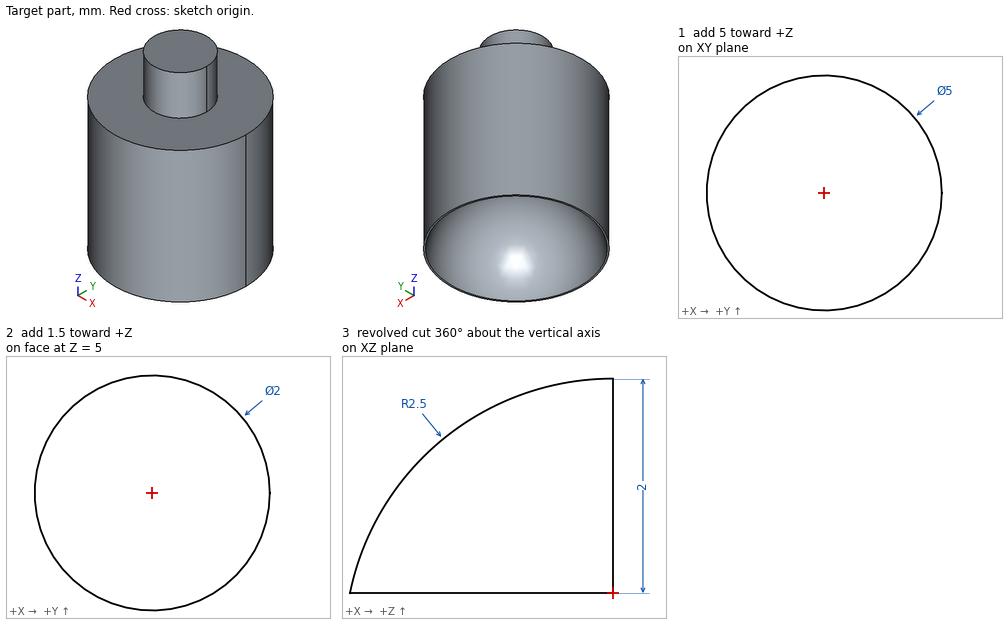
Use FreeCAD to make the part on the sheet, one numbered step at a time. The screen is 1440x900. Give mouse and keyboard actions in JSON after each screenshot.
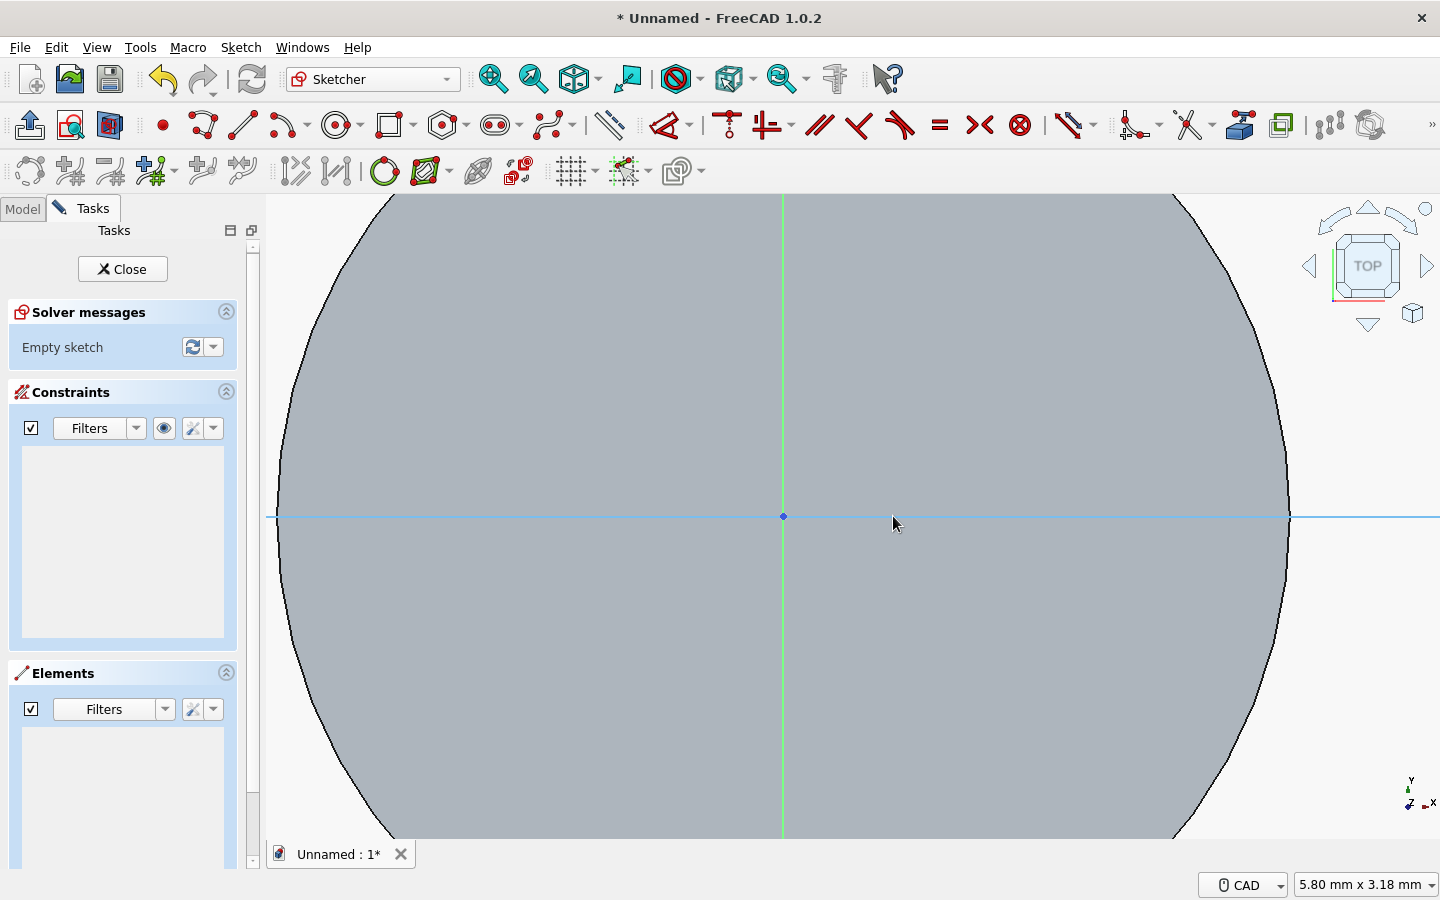
{"action": "left_click", "coordinate": [336, 126]}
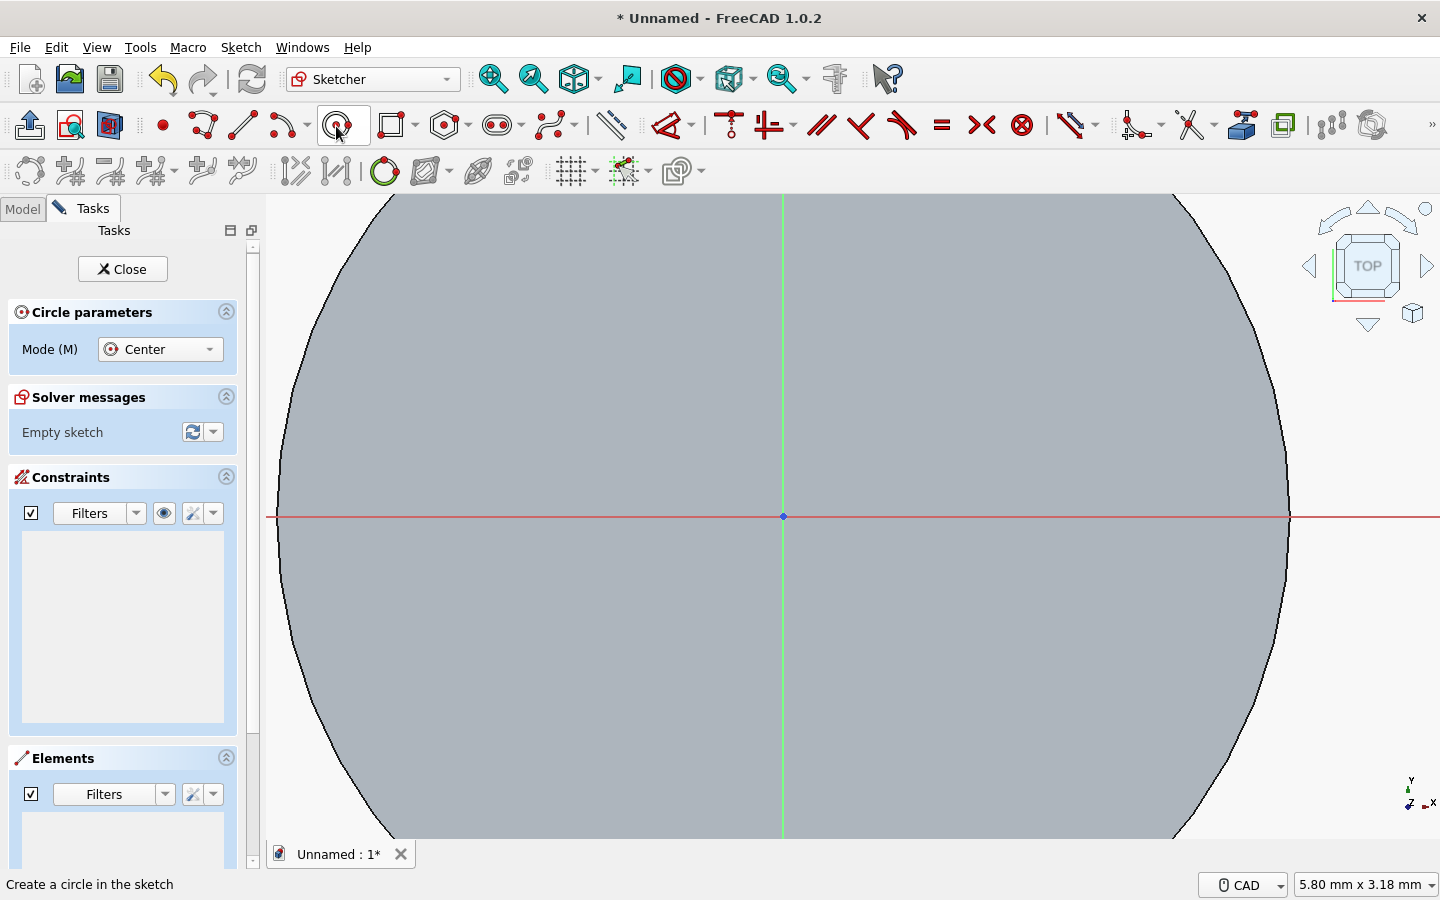
{"action": "left_click", "coordinate": [783, 516]}
{"action": "mouse_move", "coordinate": [927, 373]}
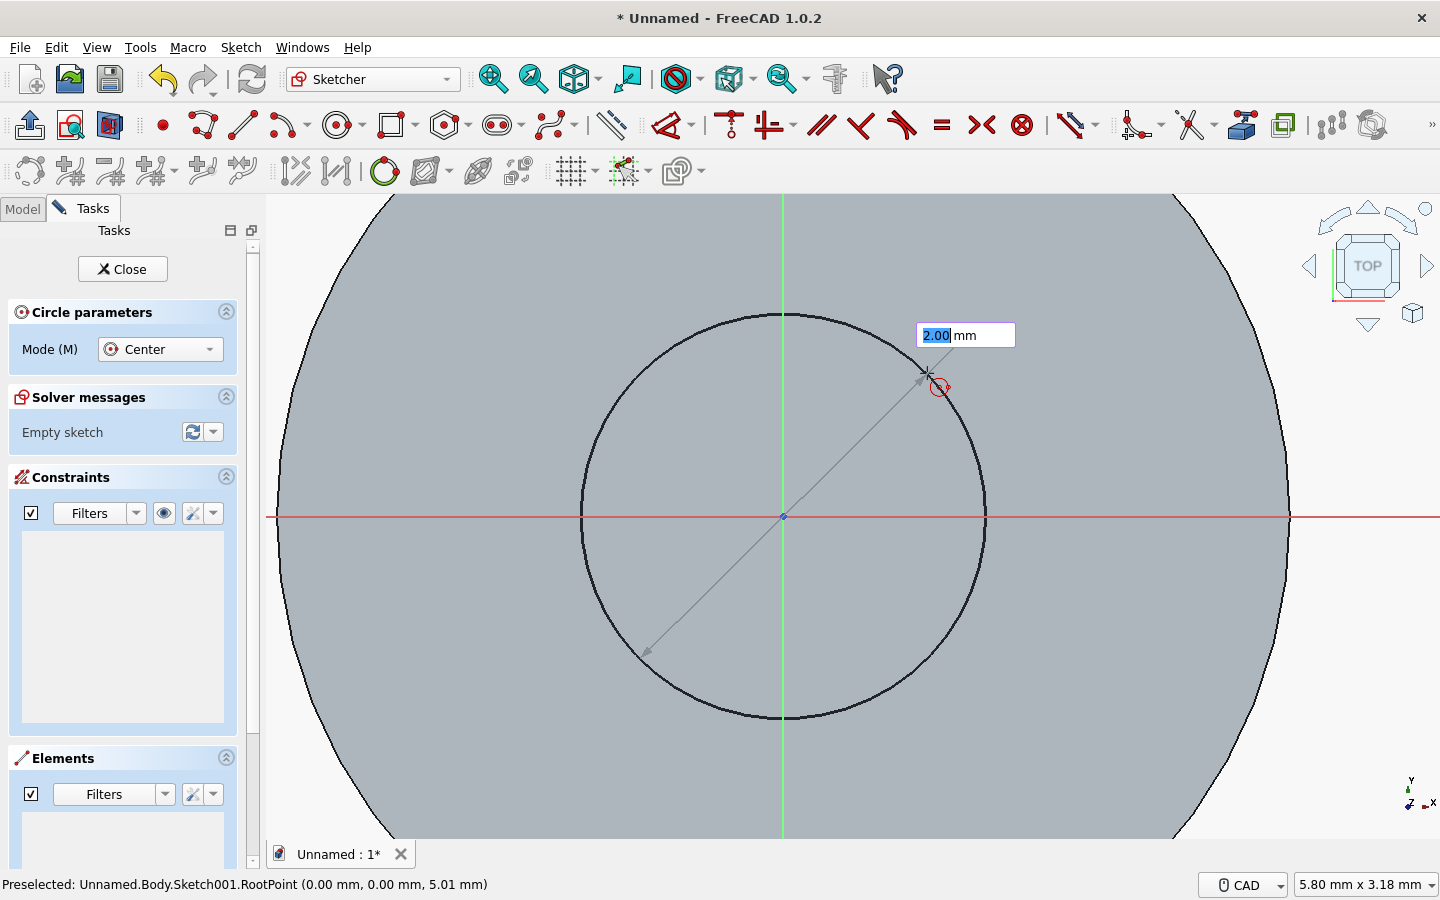
{"action": "type", "text": "2"}
{"action": "key", "text": "Return"}
{"action": "key", "text": "Escape"}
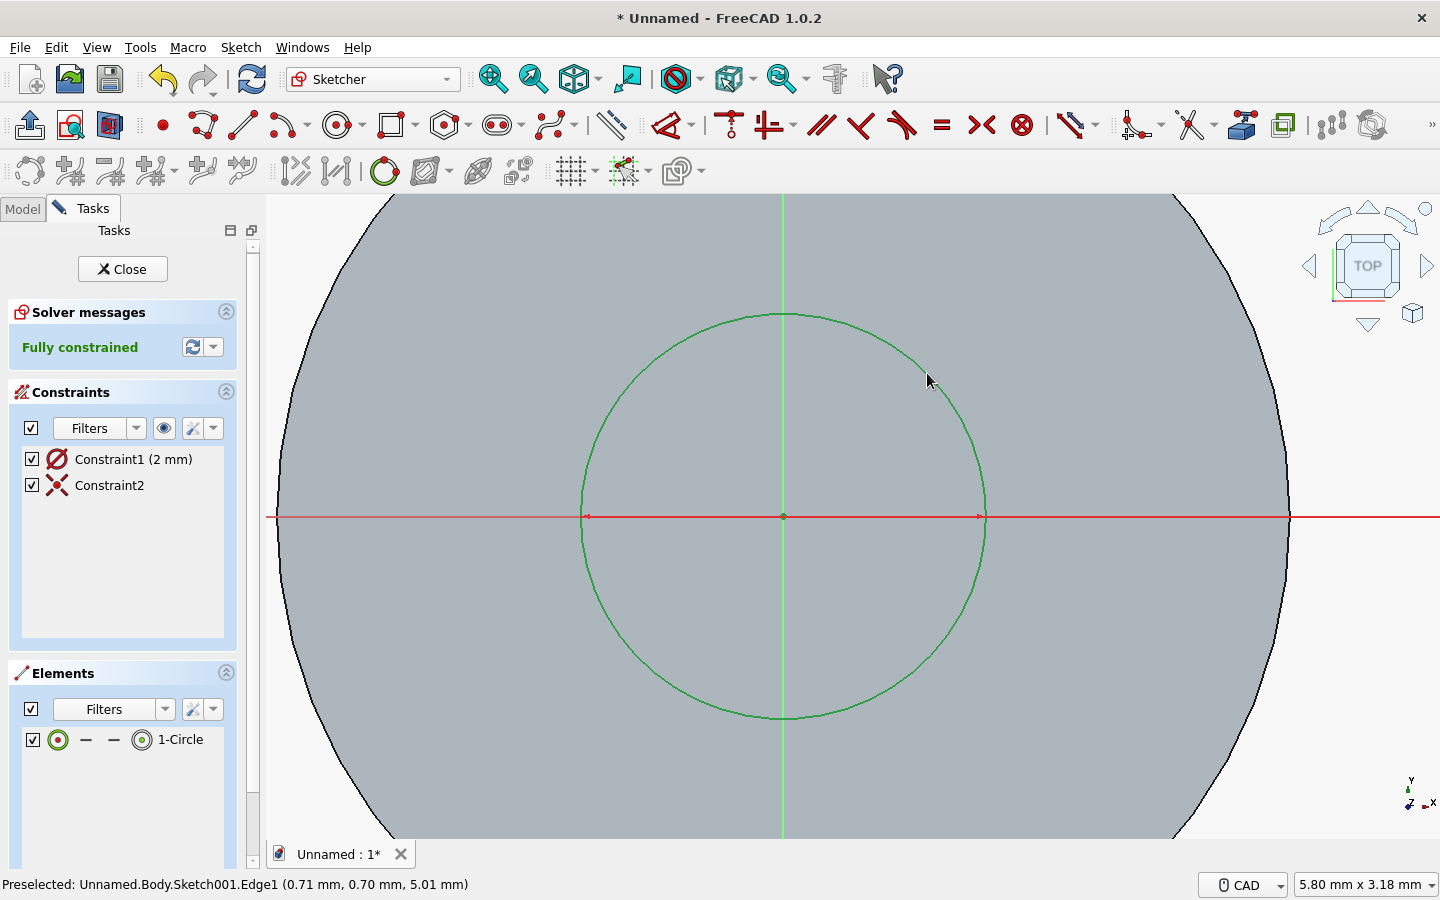
{"action": "left_click", "coordinate": [123, 269]}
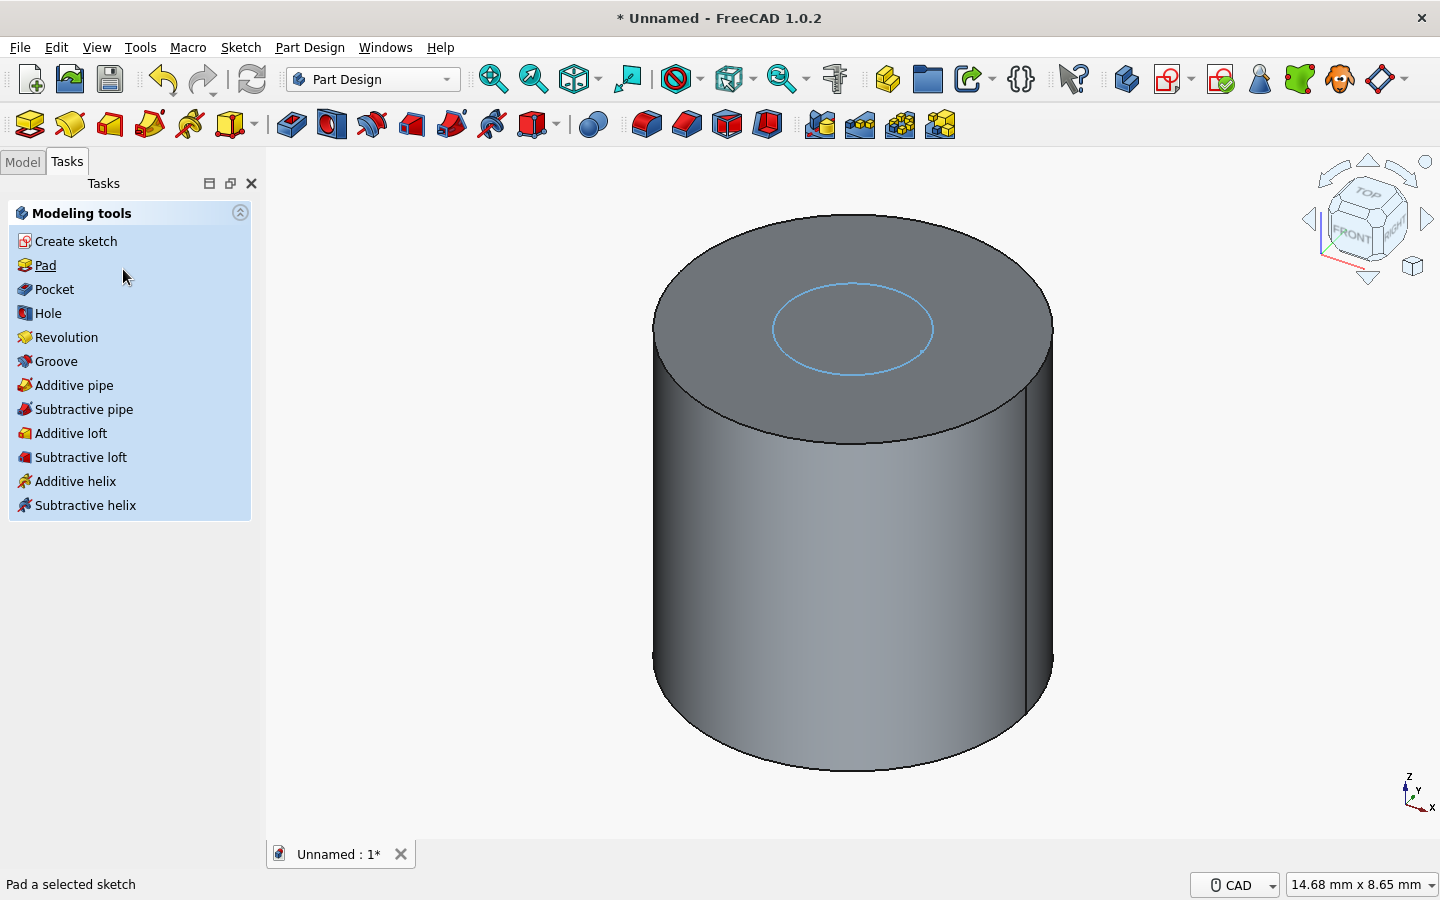
{"action": "left_click", "coordinate": [30, 124]}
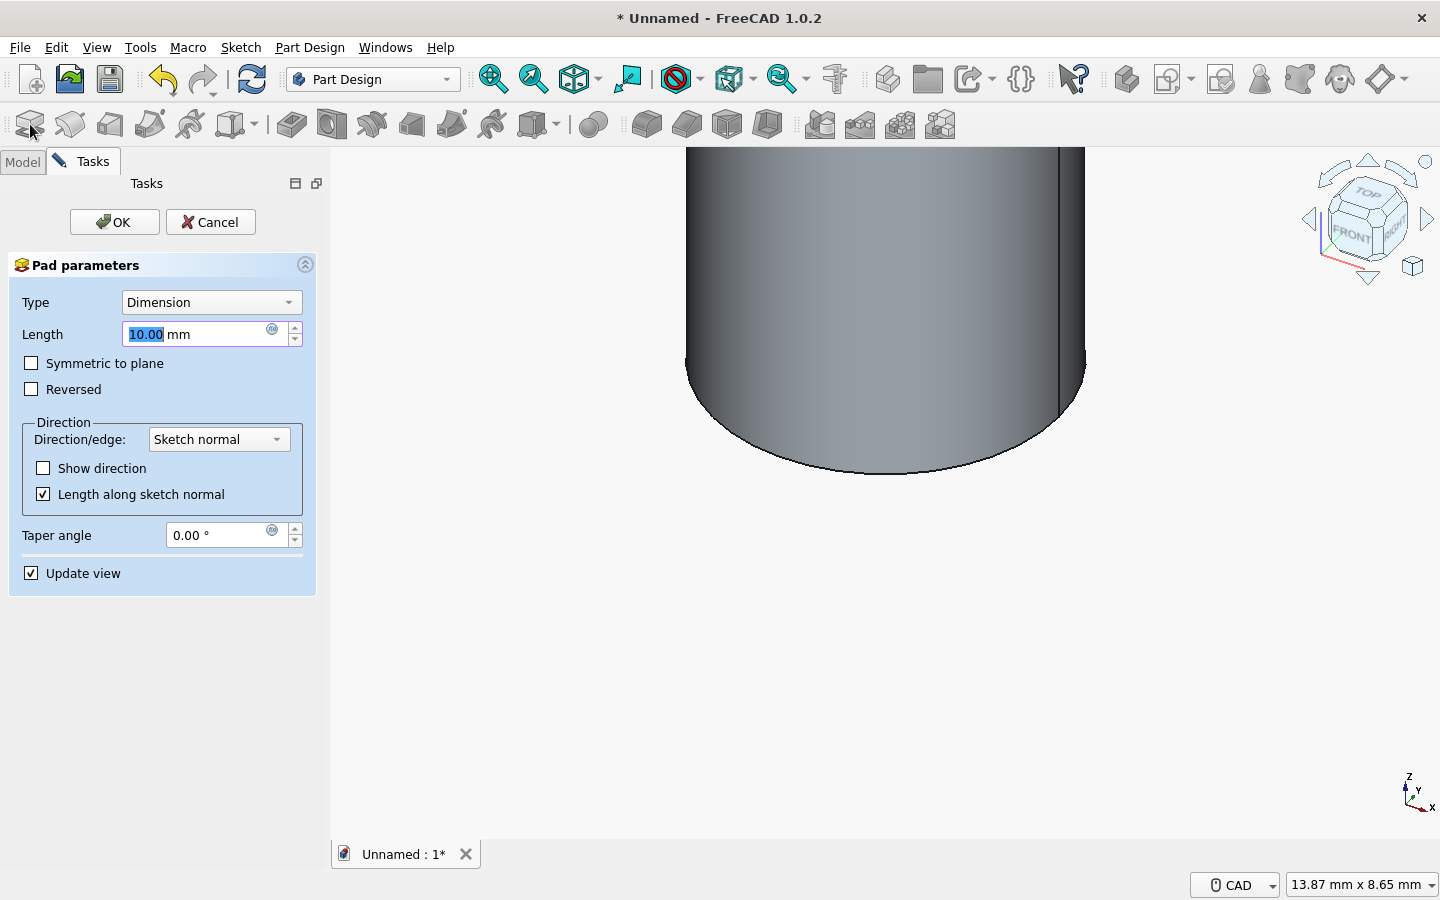
{"action": "type", "text": "1.5"}
{"action": "key", "text": "Tab"}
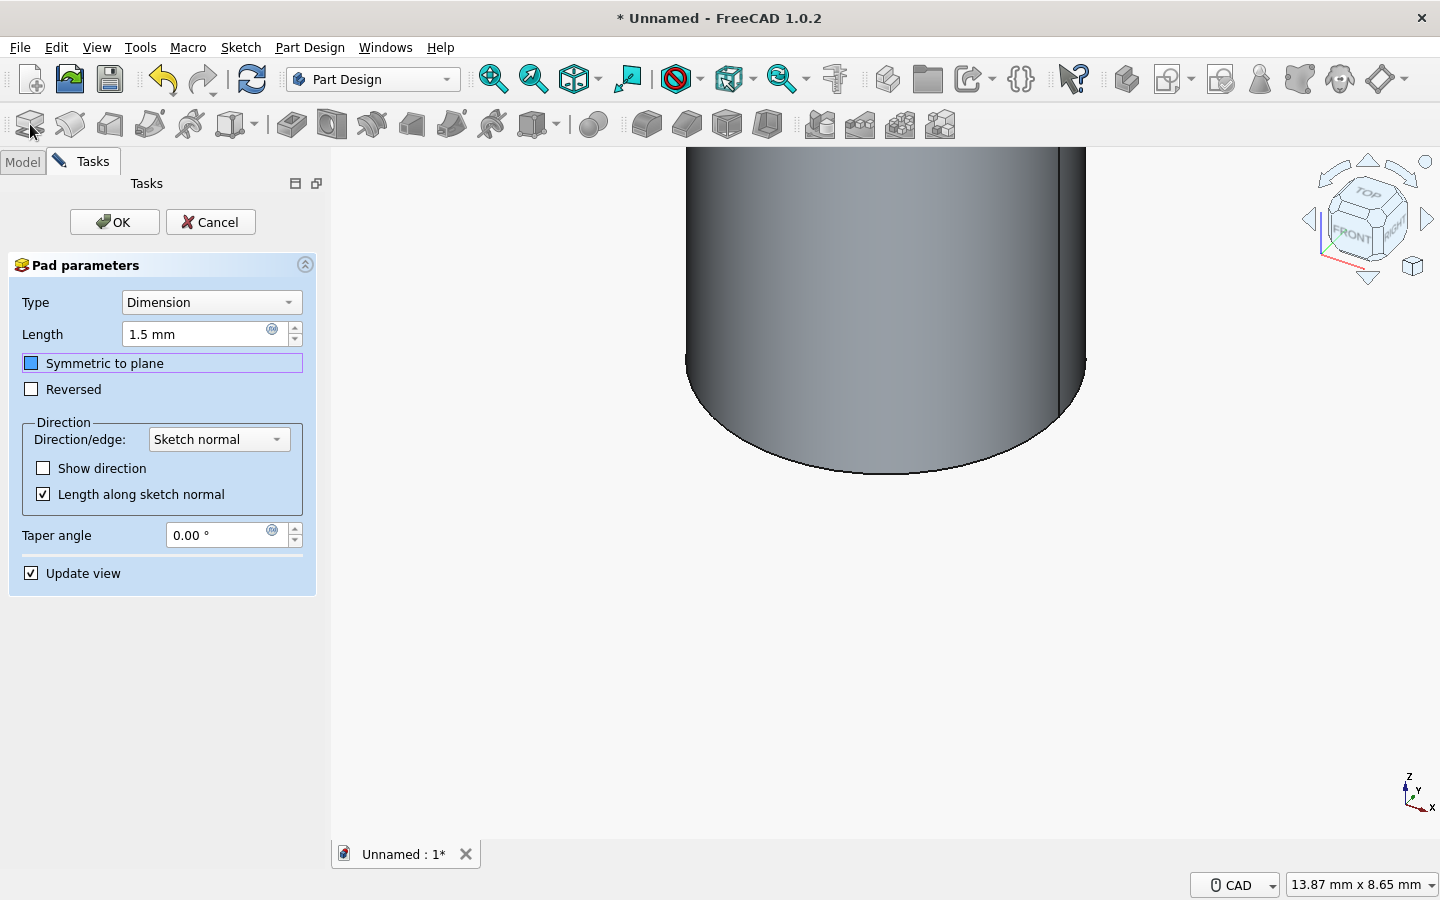
{"action": "left_click", "coordinate": [115, 222]}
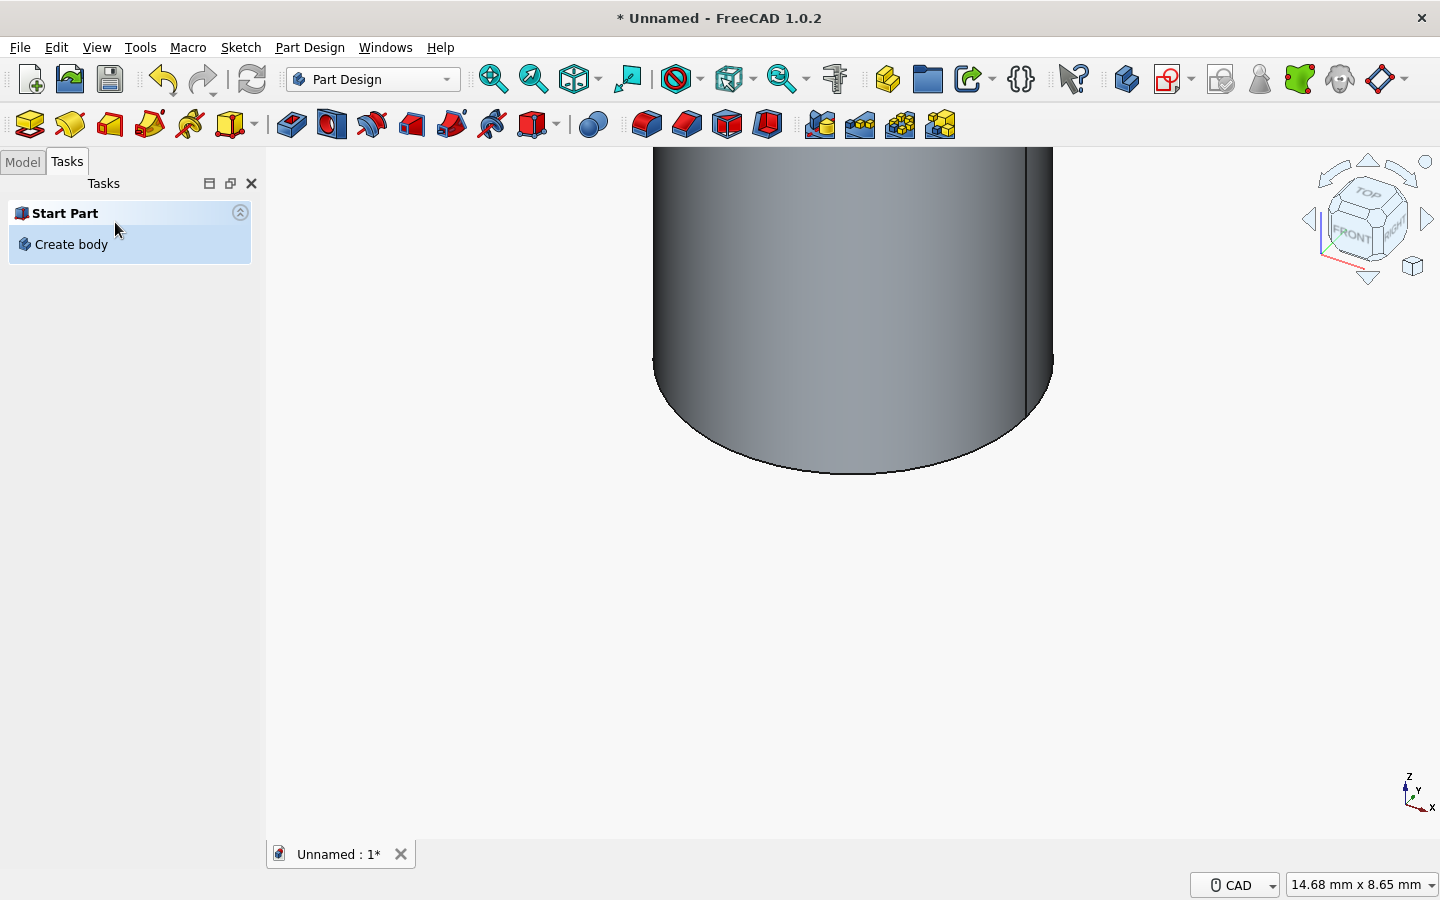
{"action": "left_click", "coordinate": [494, 80]}